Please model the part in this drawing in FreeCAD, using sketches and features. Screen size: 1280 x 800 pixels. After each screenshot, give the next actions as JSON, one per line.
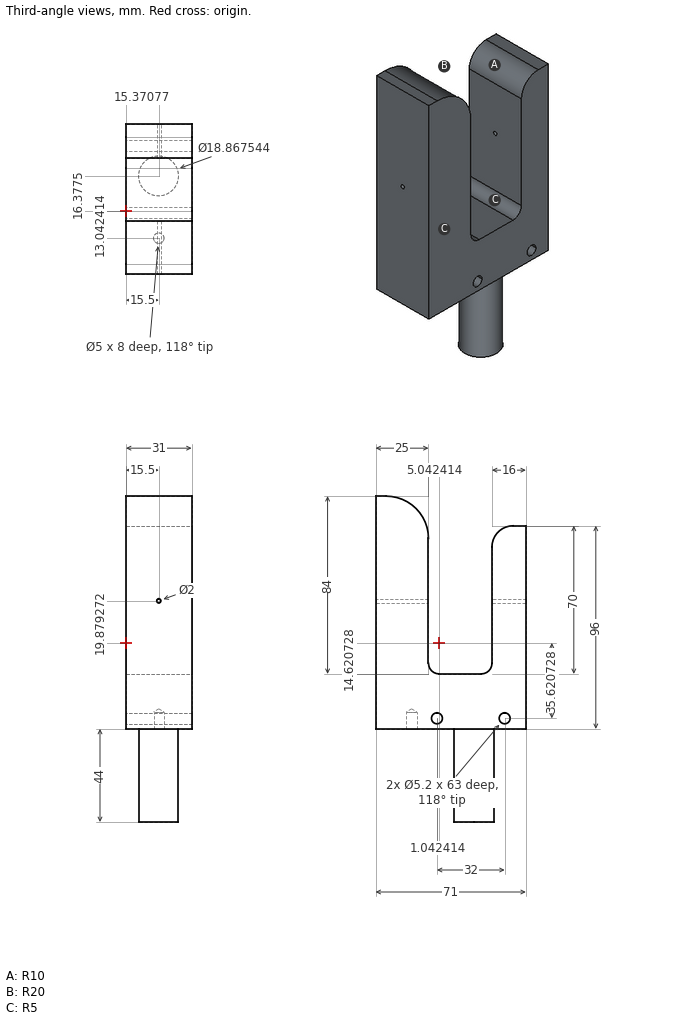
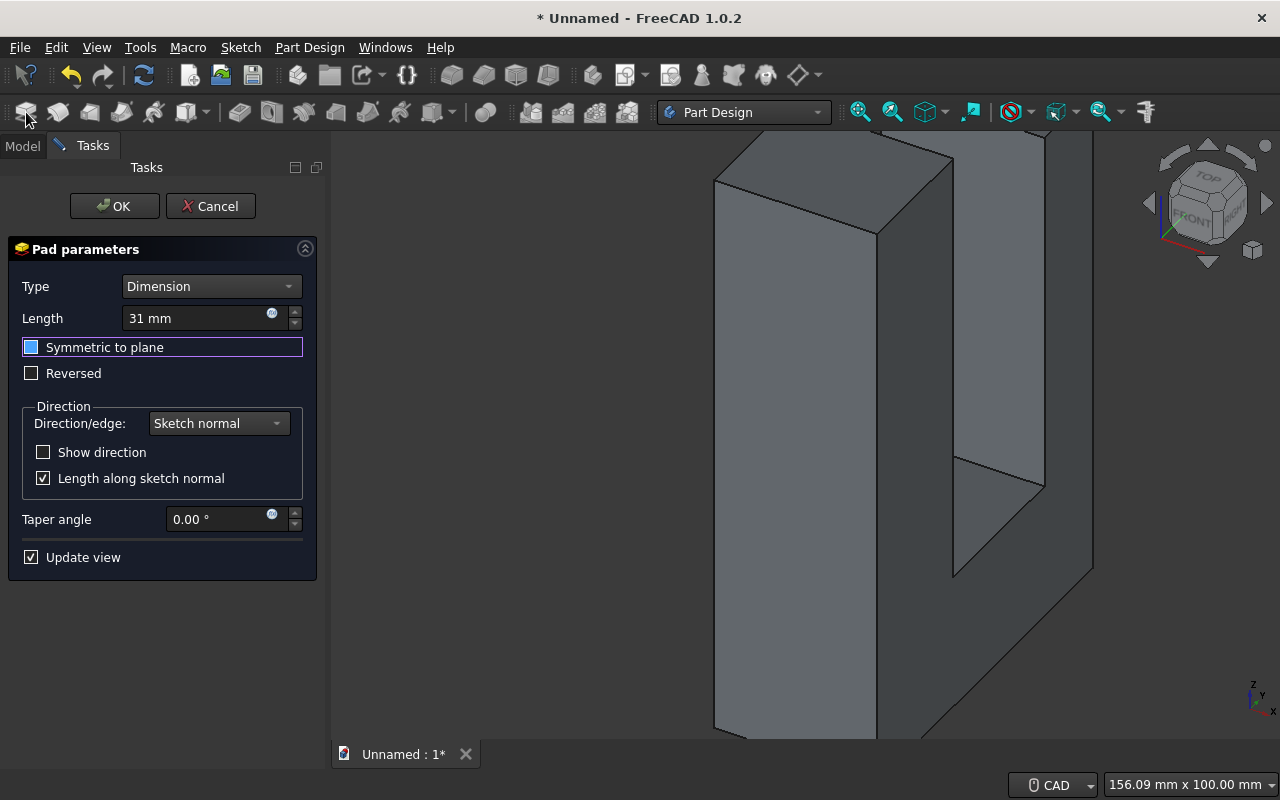
{"action": "left_click", "coordinate": [115, 206]}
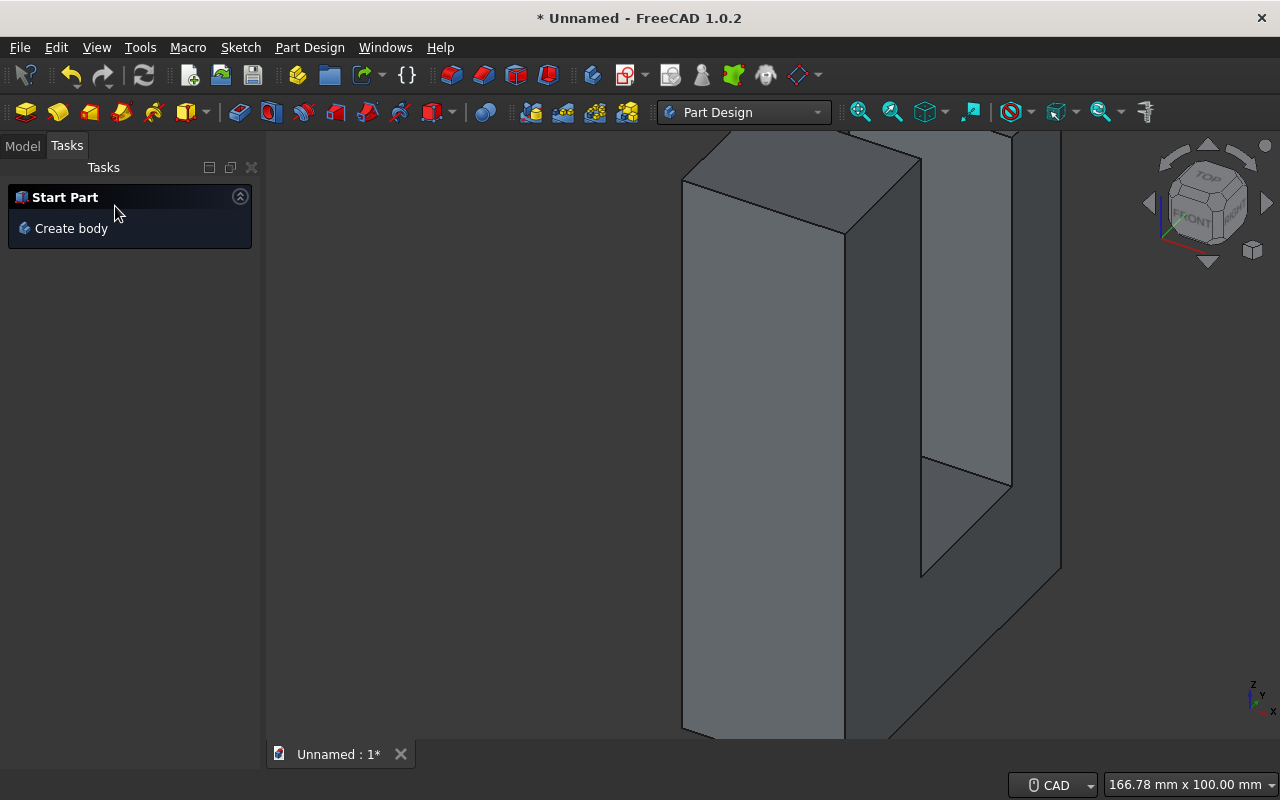
{"action": "left_click", "coordinate": [862, 112]}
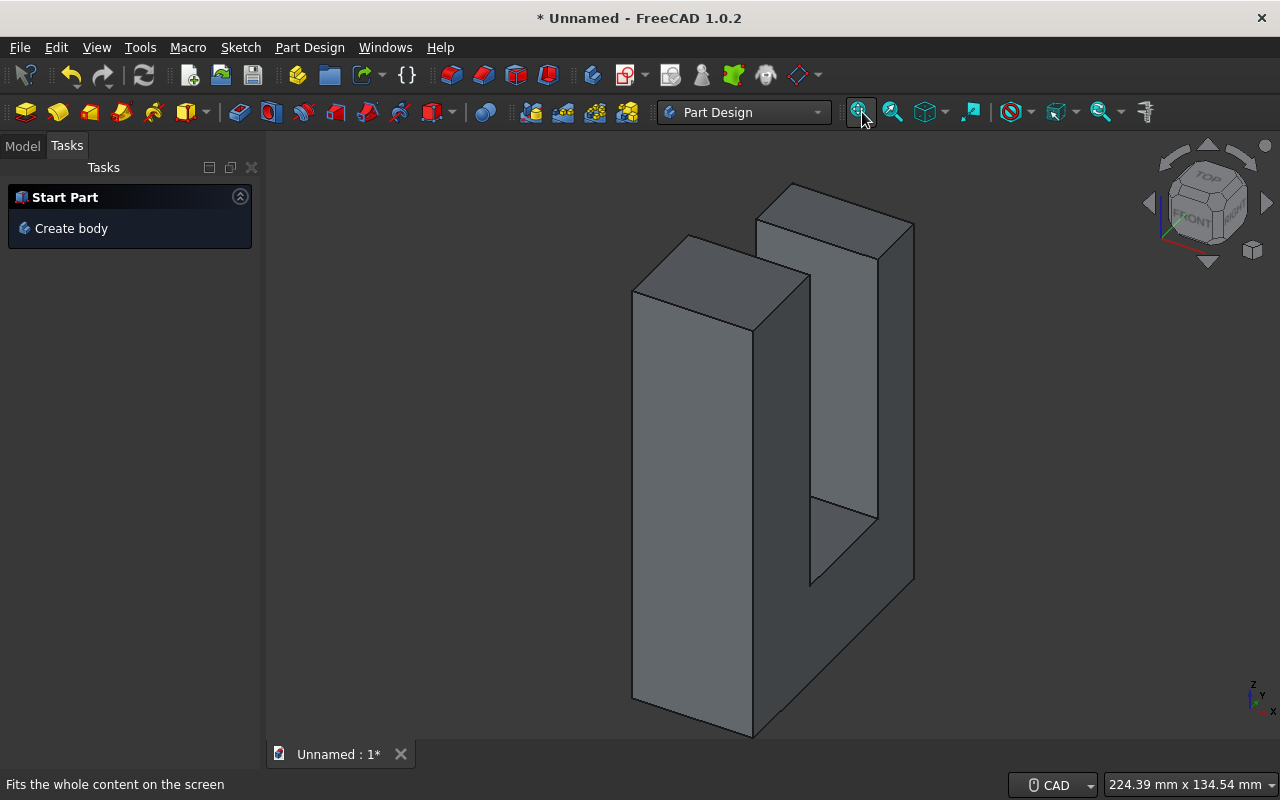
{"action": "key", "text": "4"}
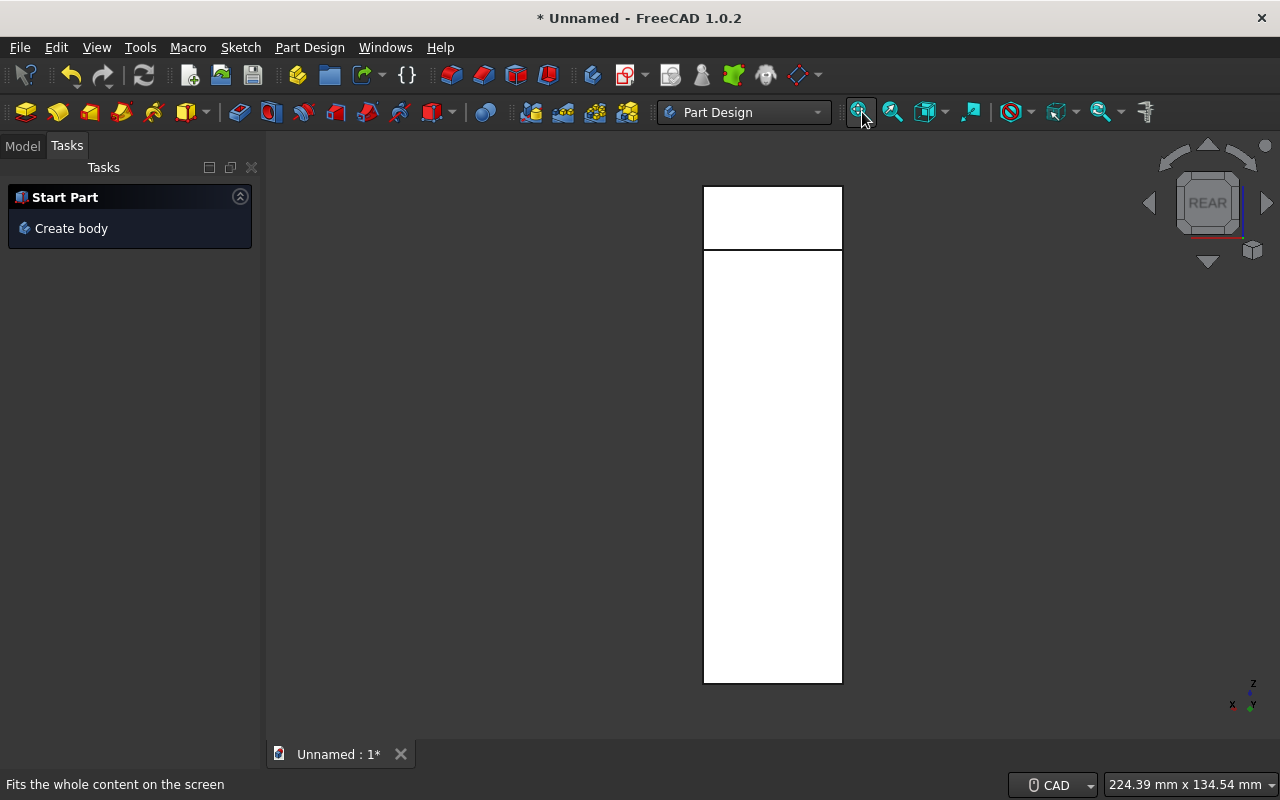
{"action": "left_click", "coordinate": [773, 528]}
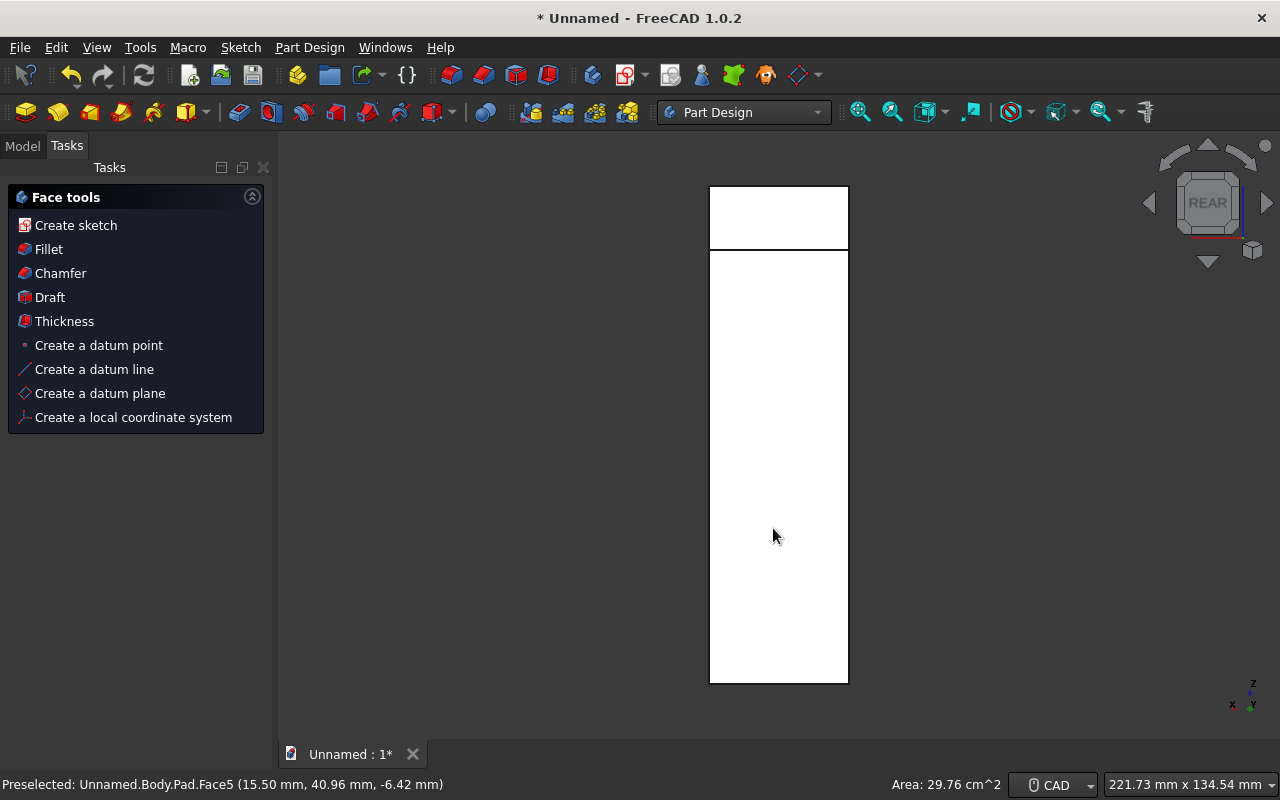
{"action": "left_click", "coordinate": [626, 76]}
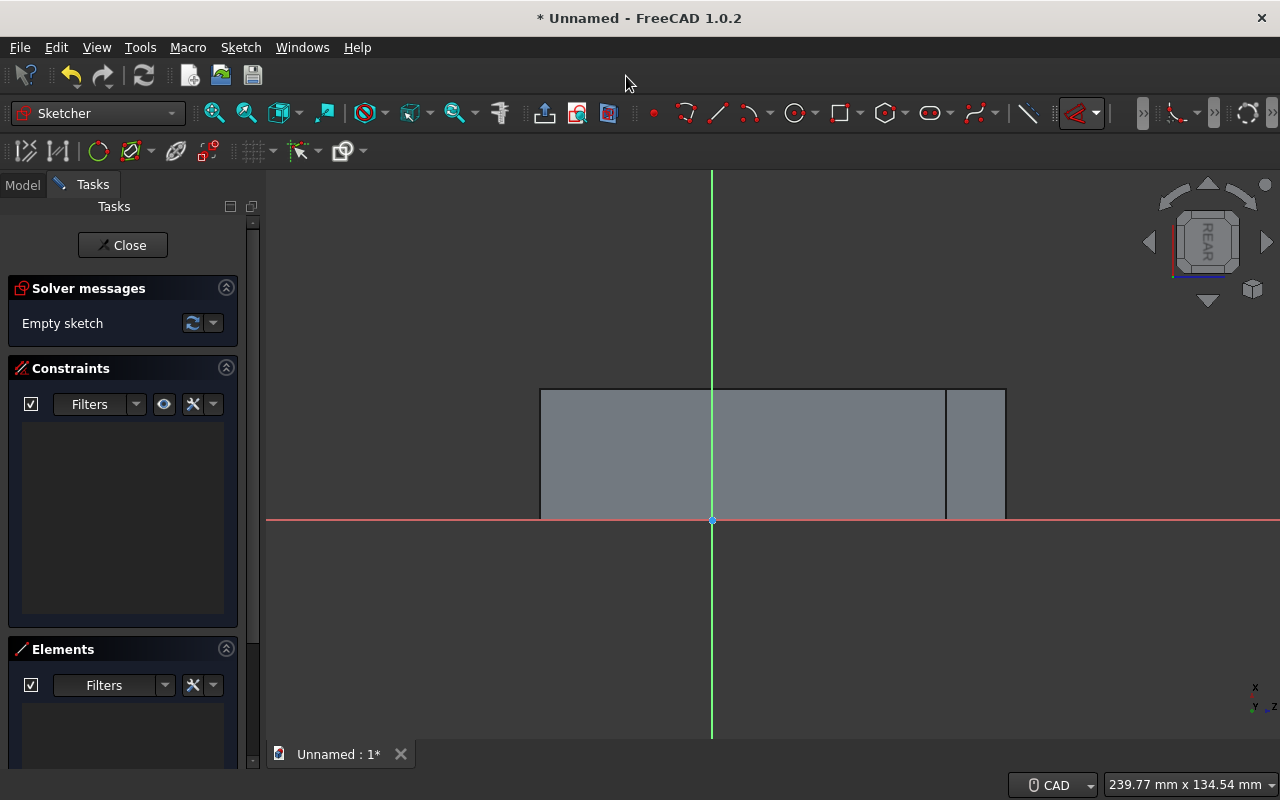
{"action": "scroll", "coordinate": [801, 455], "scroll_direction": "up", "scroll_amount": 15}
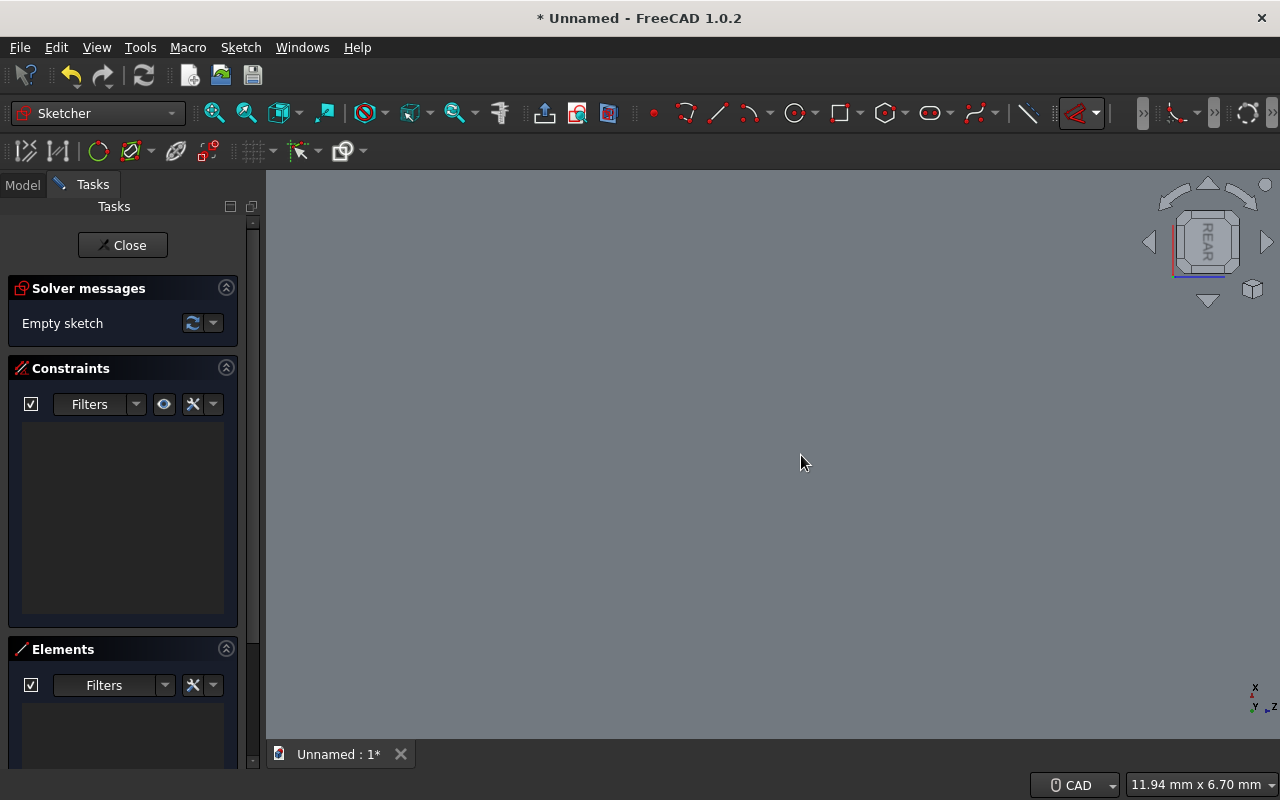
{"action": "scroll", "coordinate": [689, 420], "scroll_direction": "up", "scroll_amount": 4}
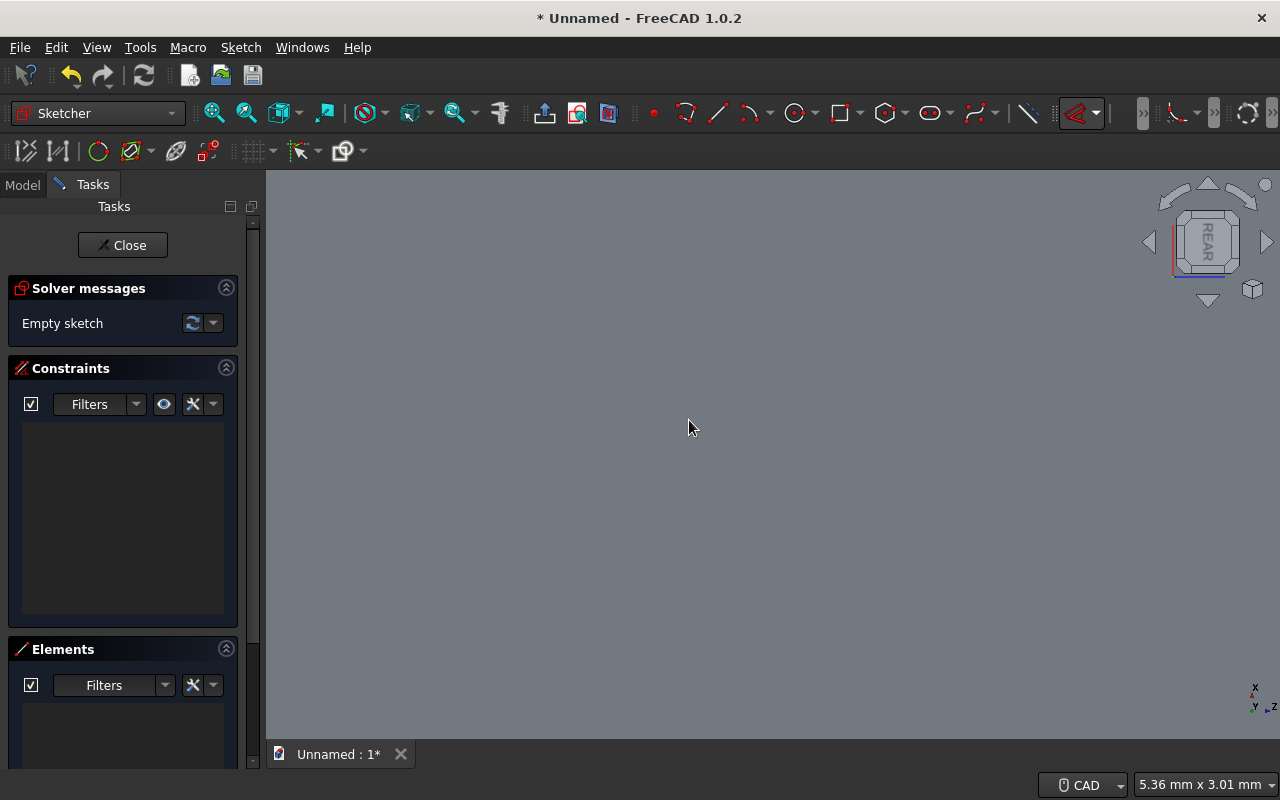
{"action": "left_click", "coordinate": [796, 114]}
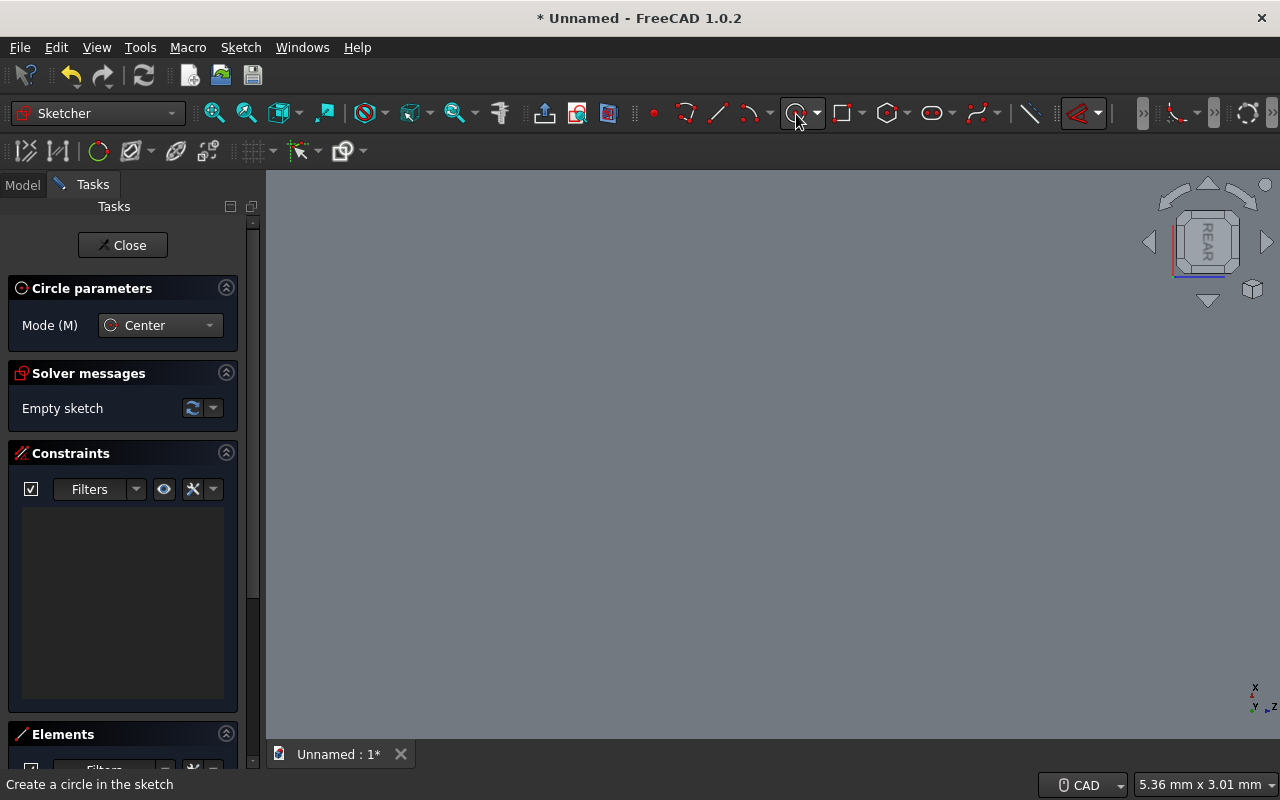
{"action": "left_click", "coordinate": [703, 454]}
{"action": "mouse_move", "coordinate": [837, 320]}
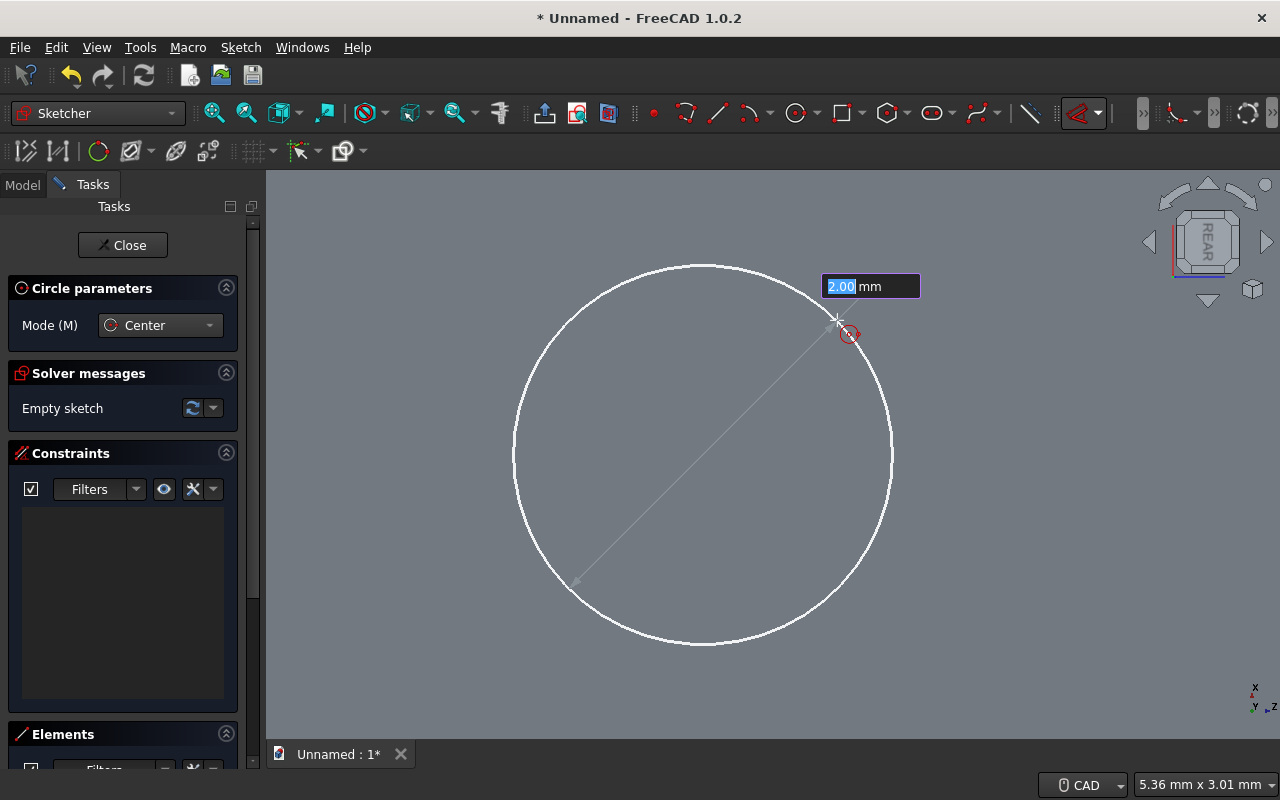
{"action": "type", "text": "2"}
{"action": "key", "text": "Return"}
{"action": "key", "text": "Escape"}